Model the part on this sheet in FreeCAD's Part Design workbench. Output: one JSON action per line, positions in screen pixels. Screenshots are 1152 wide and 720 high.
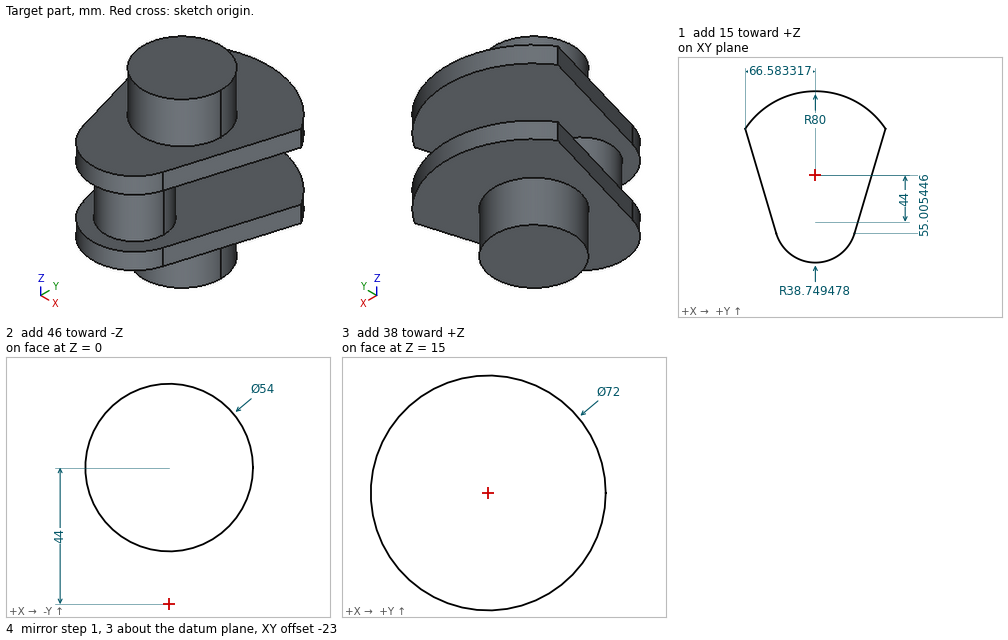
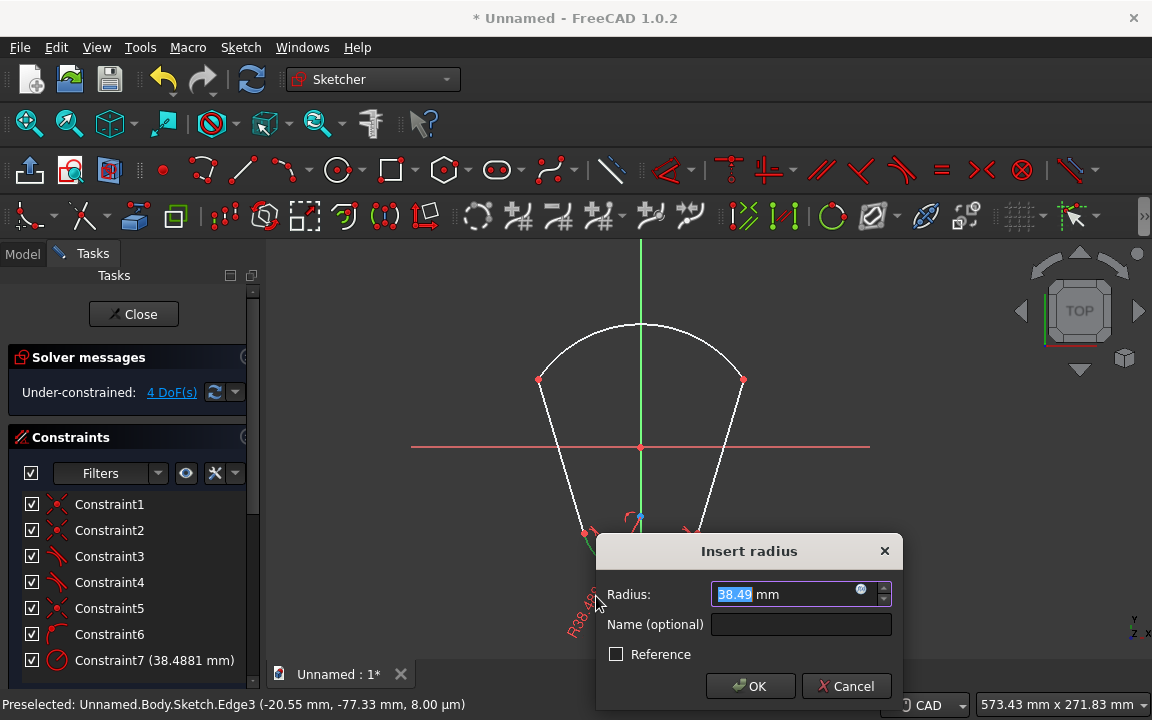
{"action": "type", "text": "38.749478"}
{"action": "key", "text": "Return"}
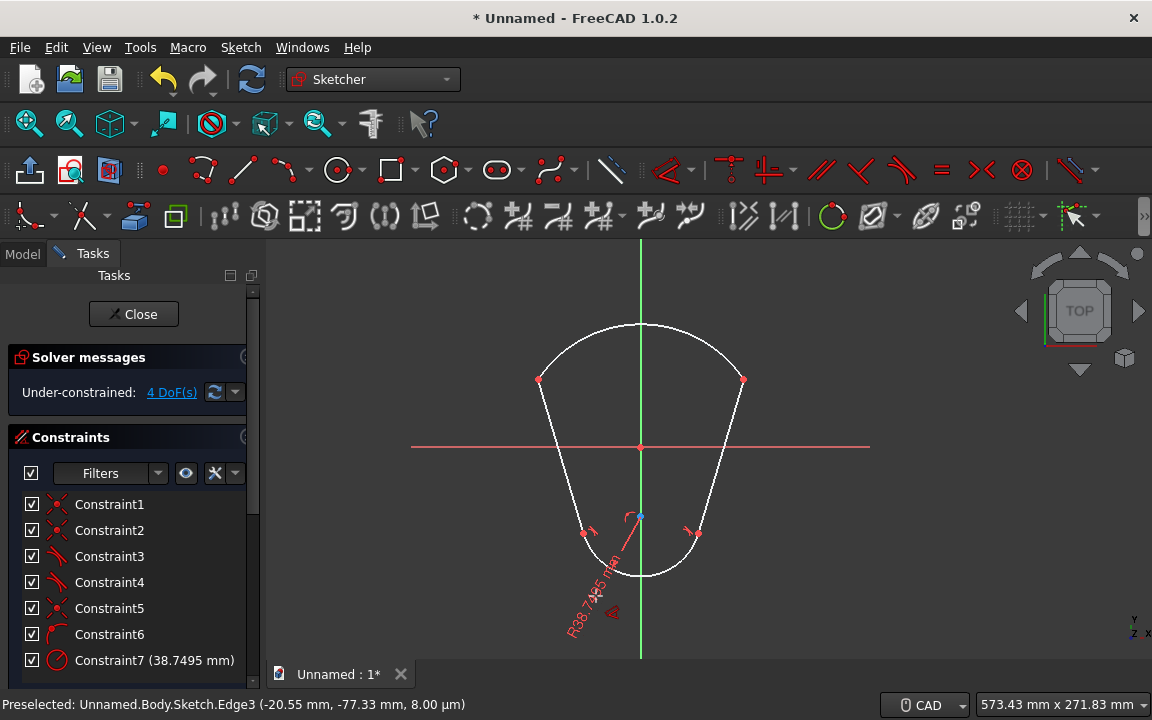
{"action": "left_click", "coordinate": [688, 334]}
{"action": "left_click", "coordinate": [700, 304]}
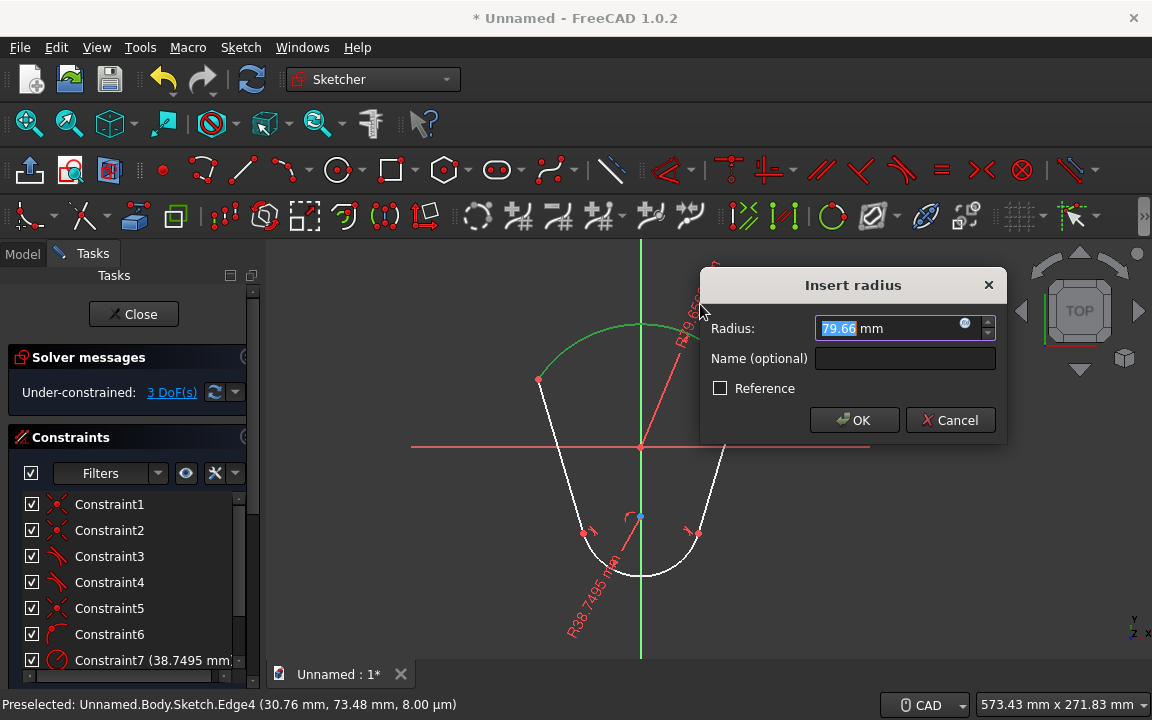
{"action": "type", "text": "80"}
{"action": "key", "text": "Return"}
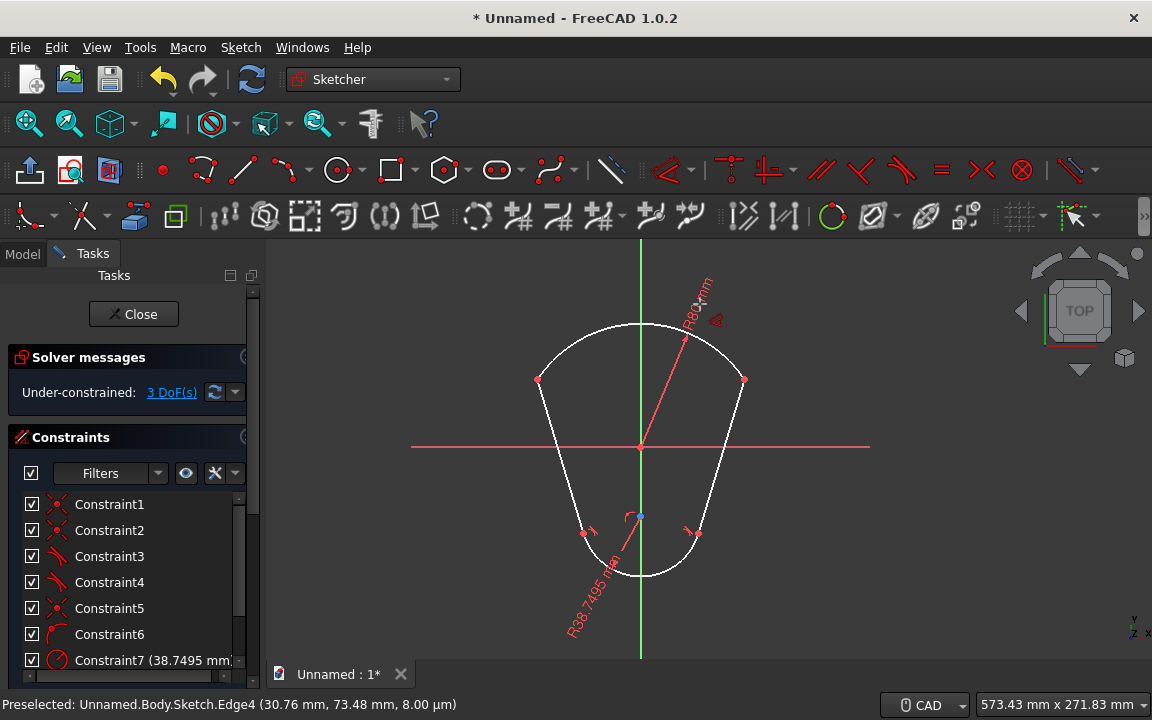
{"action": "left_click", "coordinate": [641, 517]}
{"action": "left_click", "coordinate": [675, 482]}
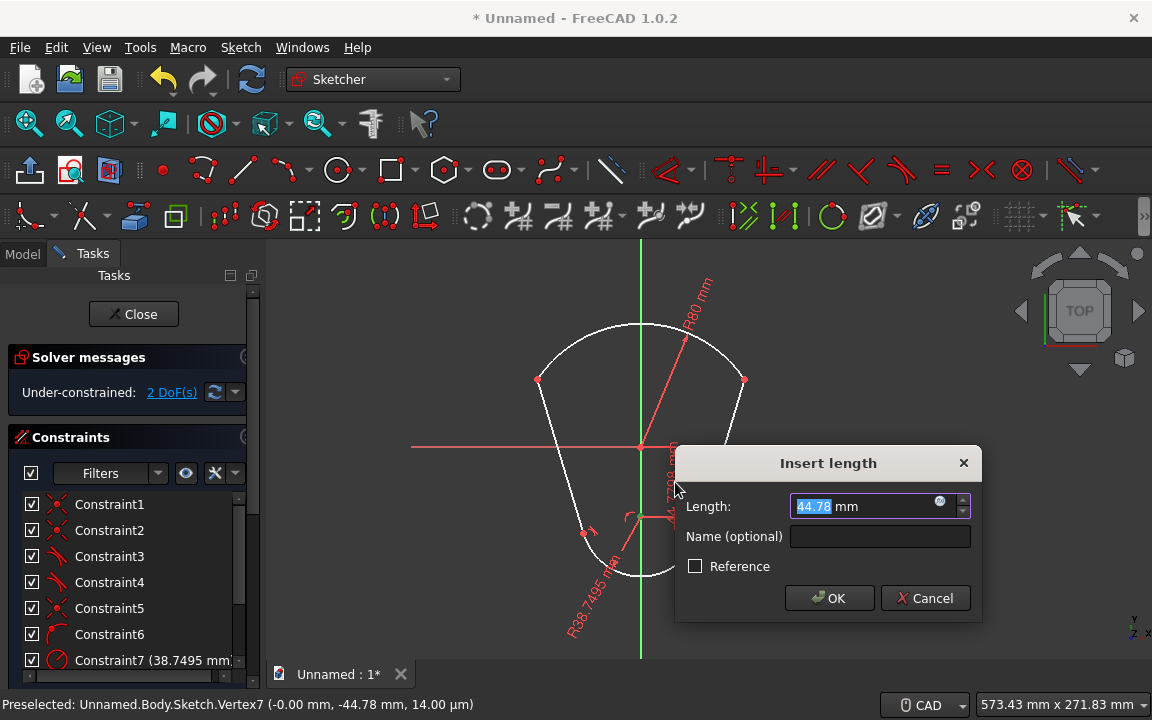
{"action": "type", "text": "44"}
{"action": "key", "text": "Return"}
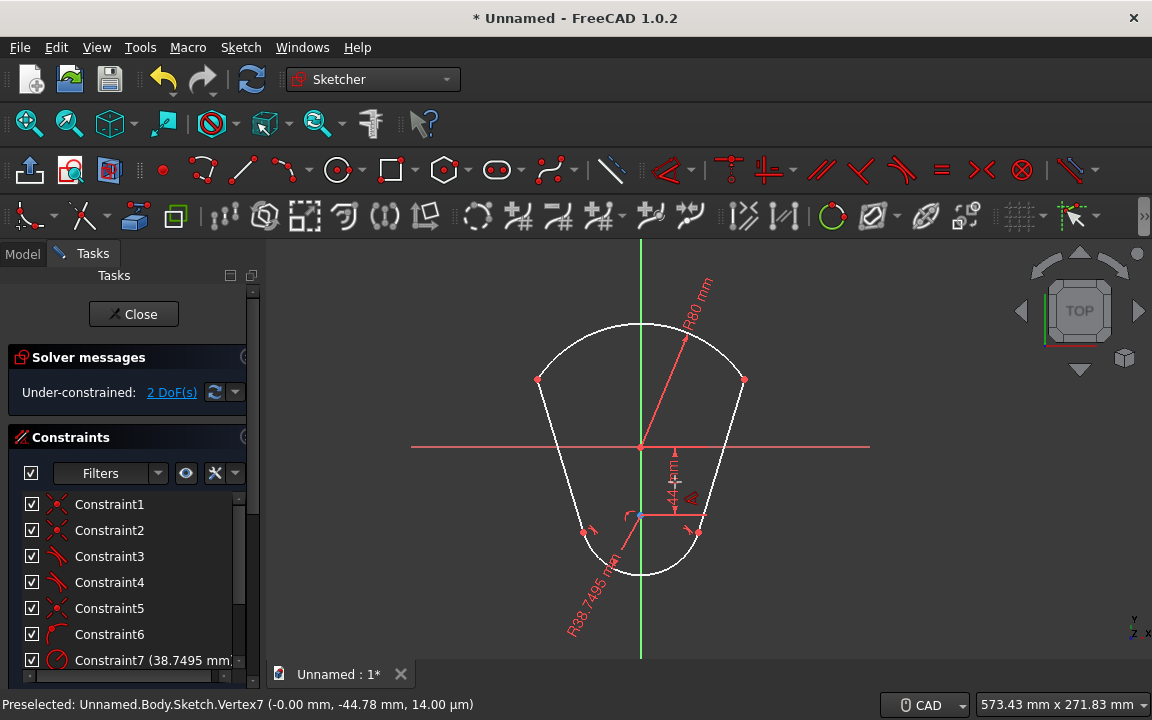
{"action": "left_click", "coordinate": [537, 380]}
{"action": "left_click", "coordinate": [613, 346]}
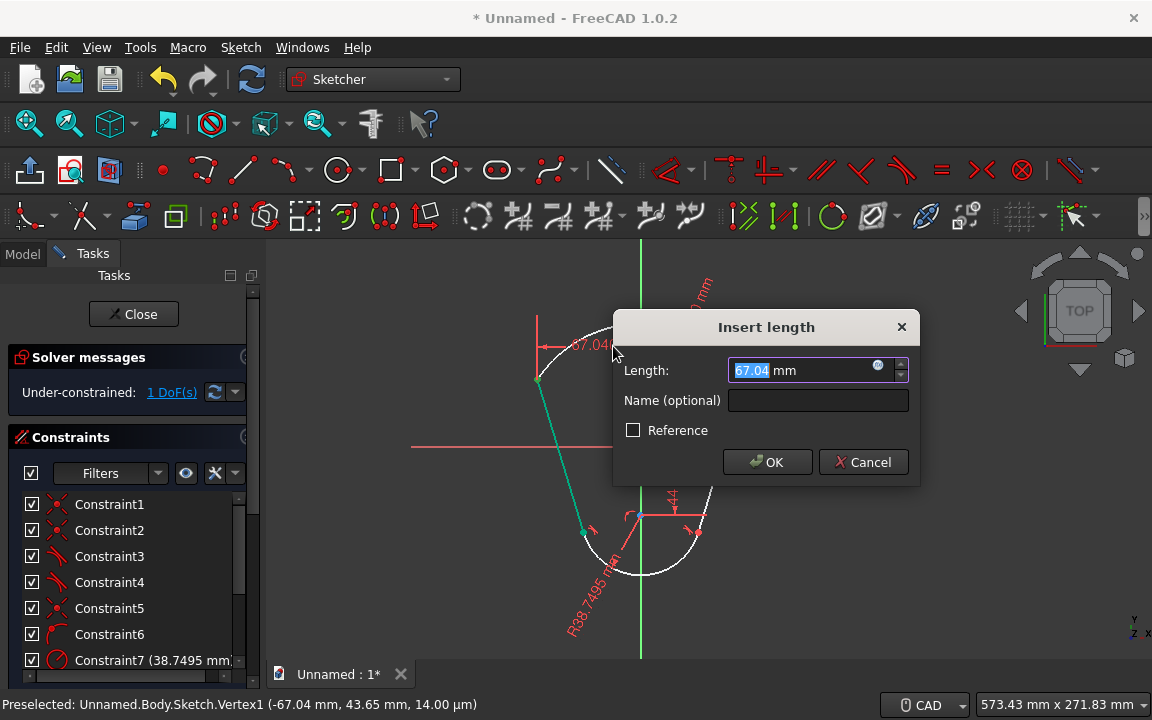
{"action": "type", "text": "66.583317"}
{"action": "key", "text": "Return"}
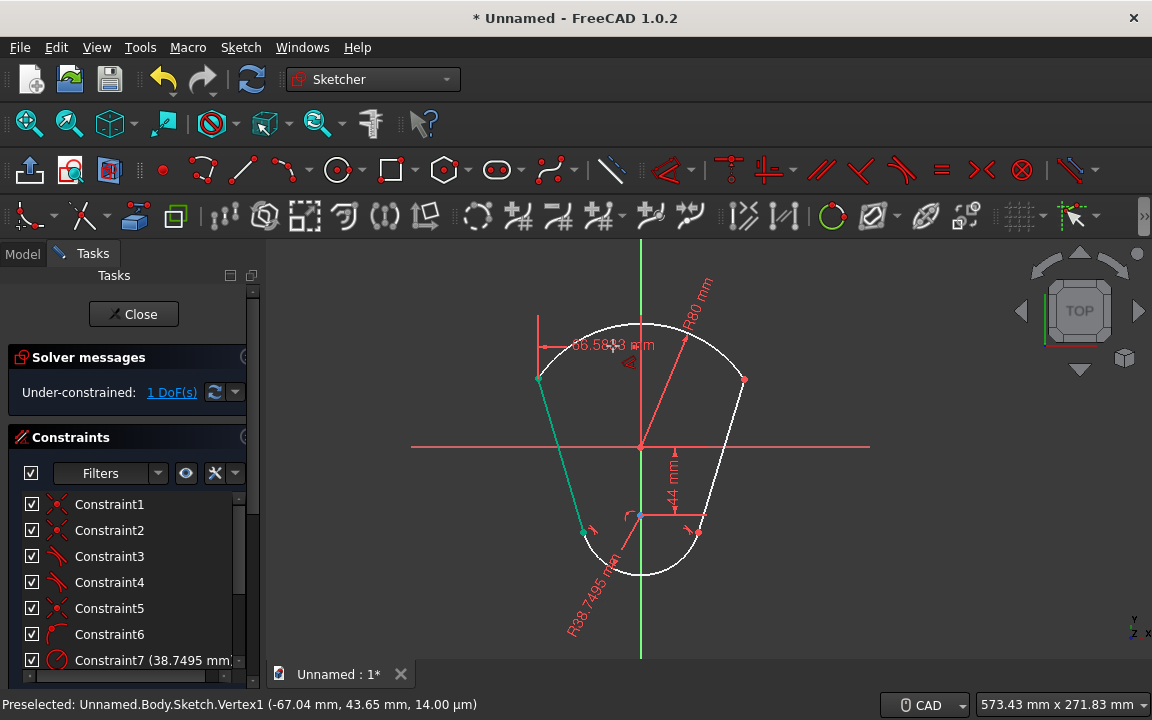
{"action": "left_click", "coordinate": [698, 533]}
{"action": "left_click", "coordinate": [732, 510]}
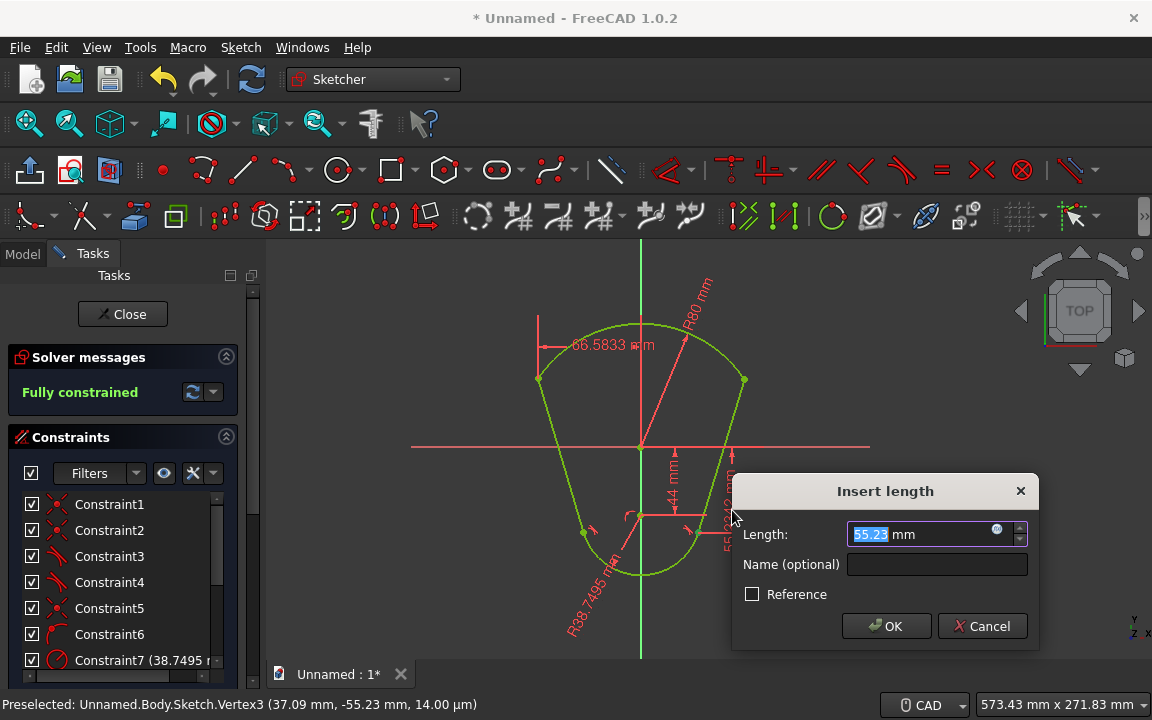
{"action": "type", "text": "55.005446"}
{"action": "key", "text": "Return"}
{"action": "key", "text": "Escape"}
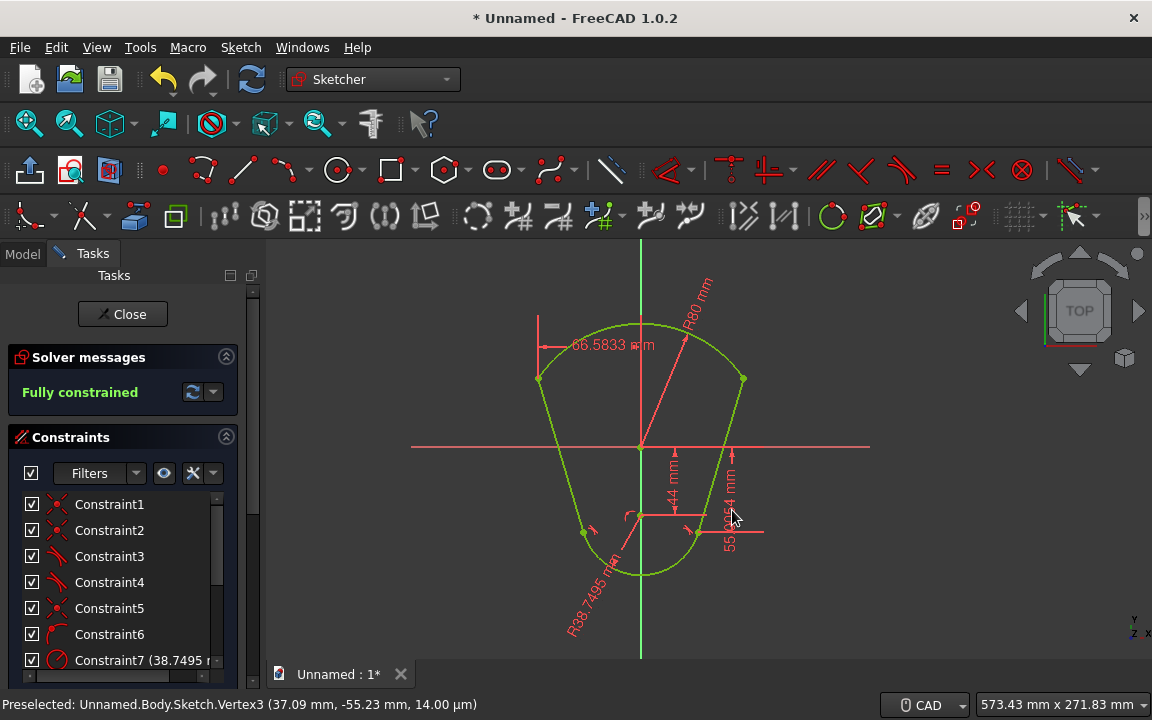
{"action": "left_click", "coordinate": [123, 314]}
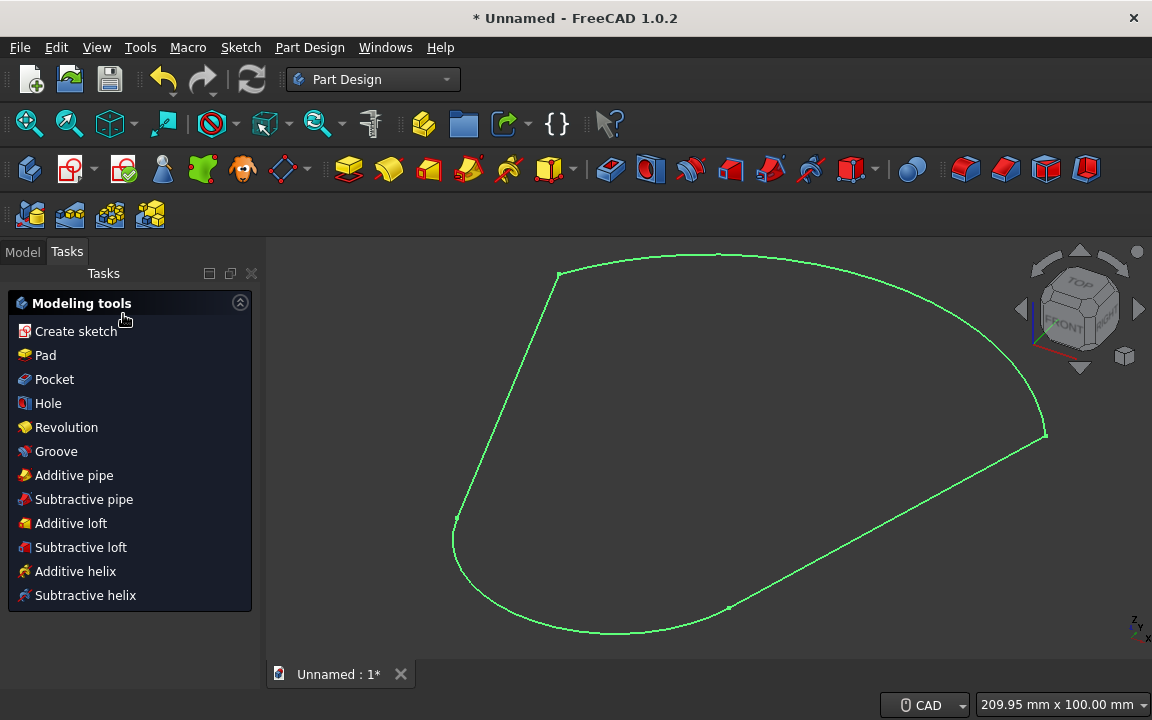
{"action": "left_click", "coordinate": [350, 170]}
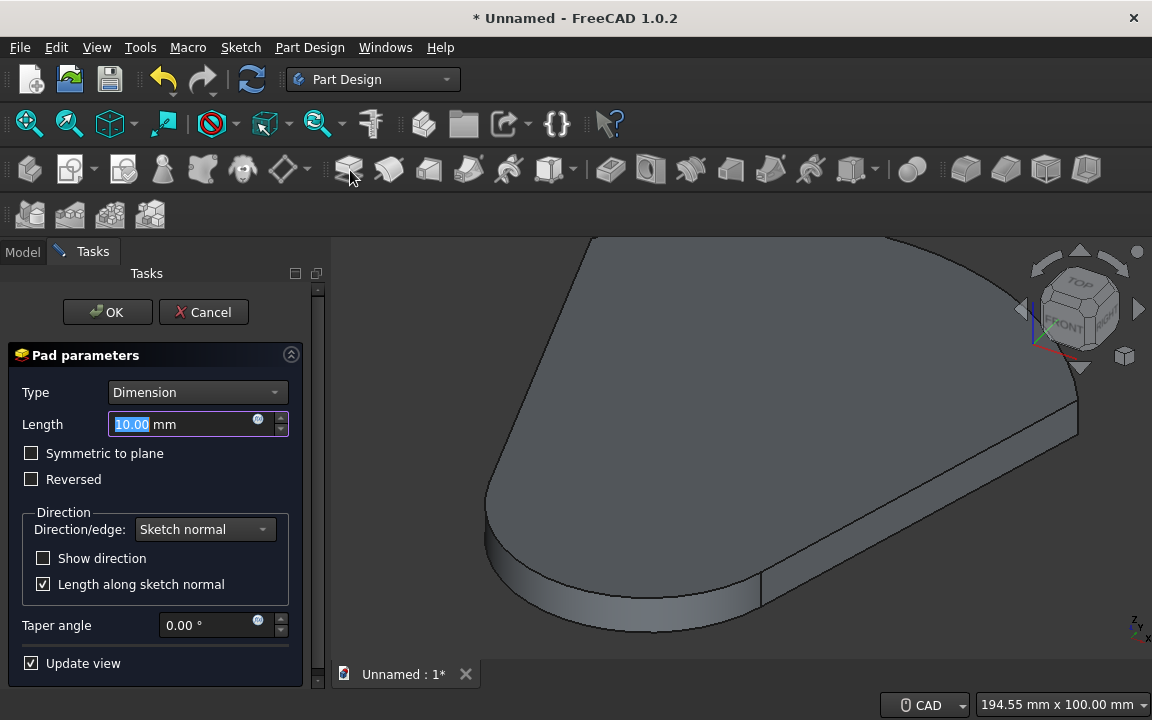
{"action": "type", "text": "15"}
{"action": "key", "text": "Tab"}